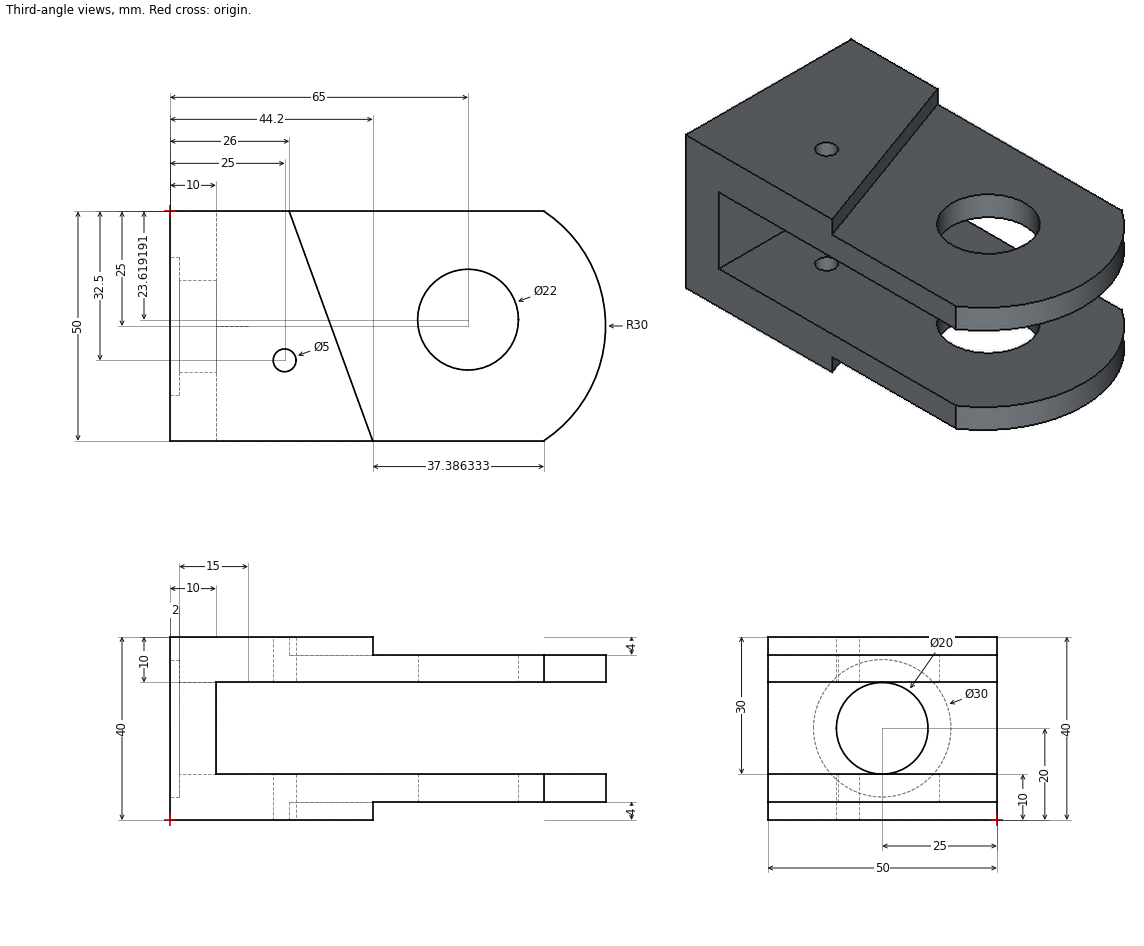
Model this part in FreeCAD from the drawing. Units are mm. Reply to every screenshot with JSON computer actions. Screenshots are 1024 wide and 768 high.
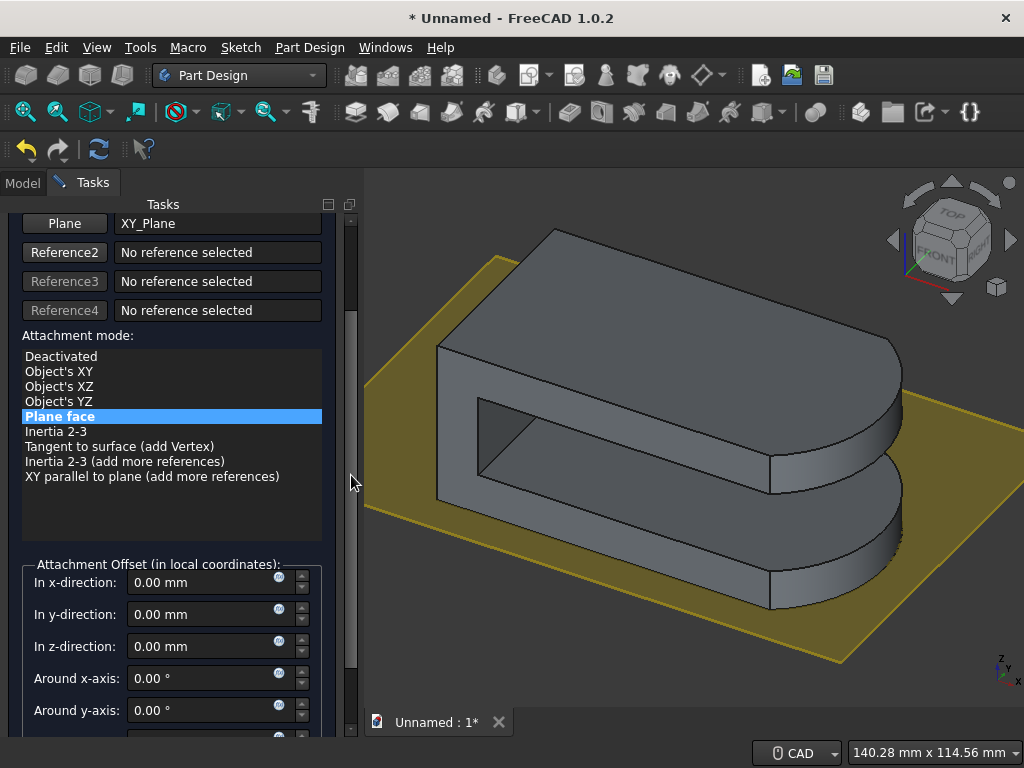
{"action": "triple_click", "coordinate": [210, 646]}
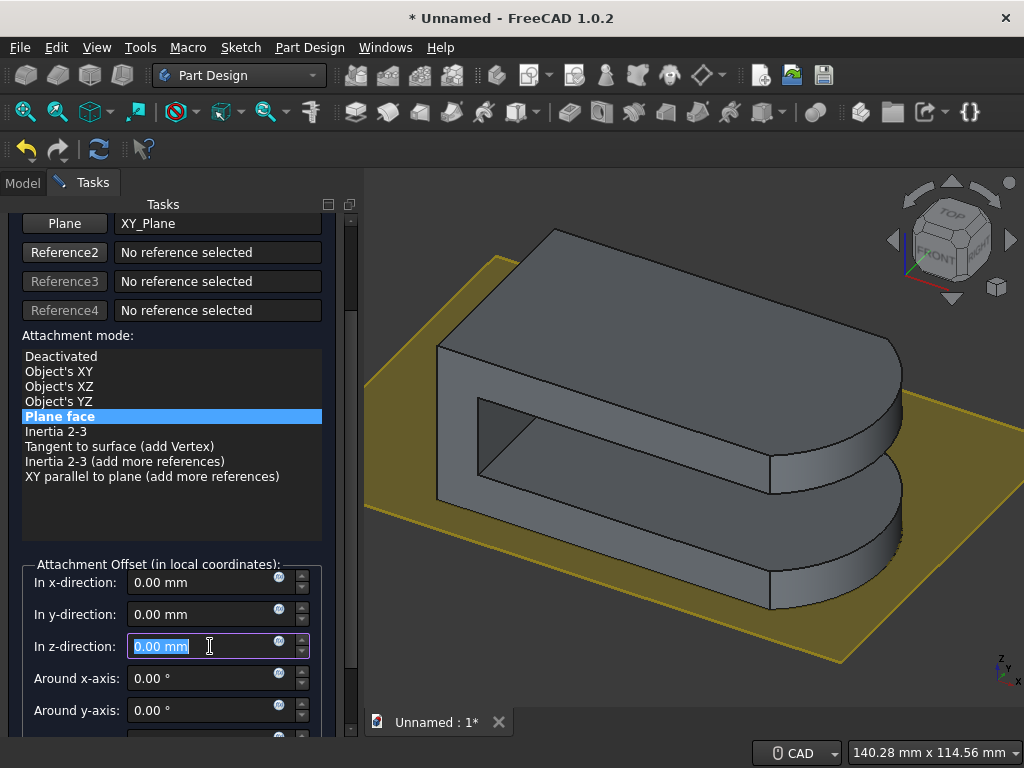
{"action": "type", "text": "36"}
{"action": "key", "text": "Tab"}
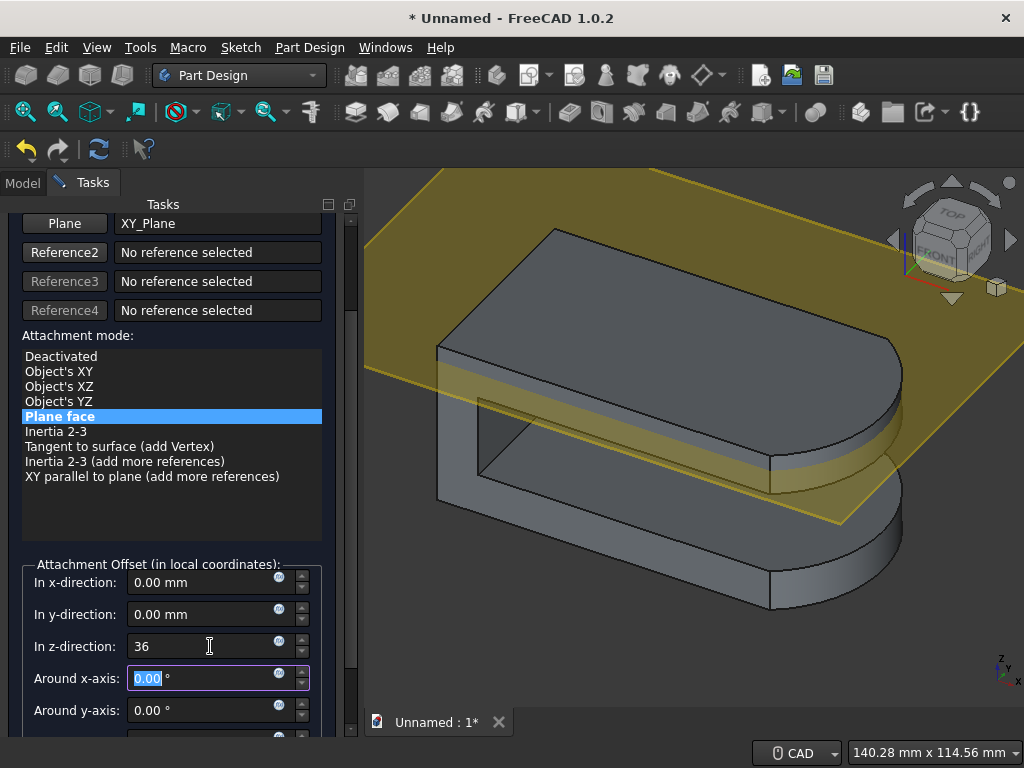
{"action": "scroll", "coordinate": [351, 475], "scroll_direction": "up", "scroll_amount": 3}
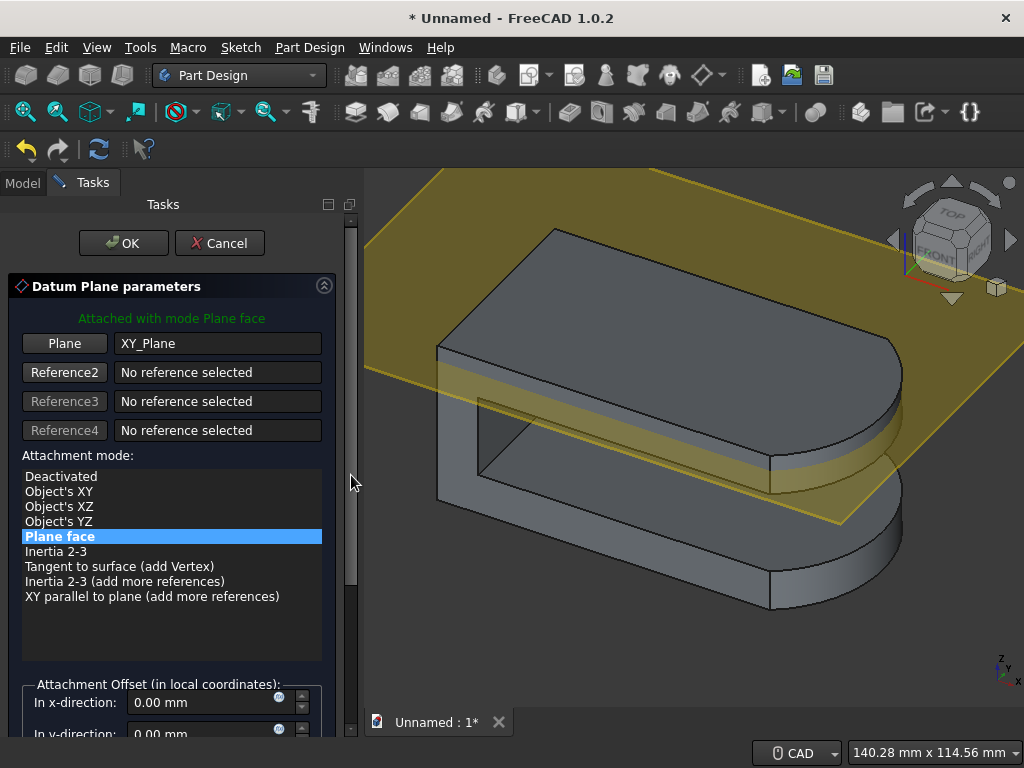
{"action": "left_click", "coordinate": [124, 243]}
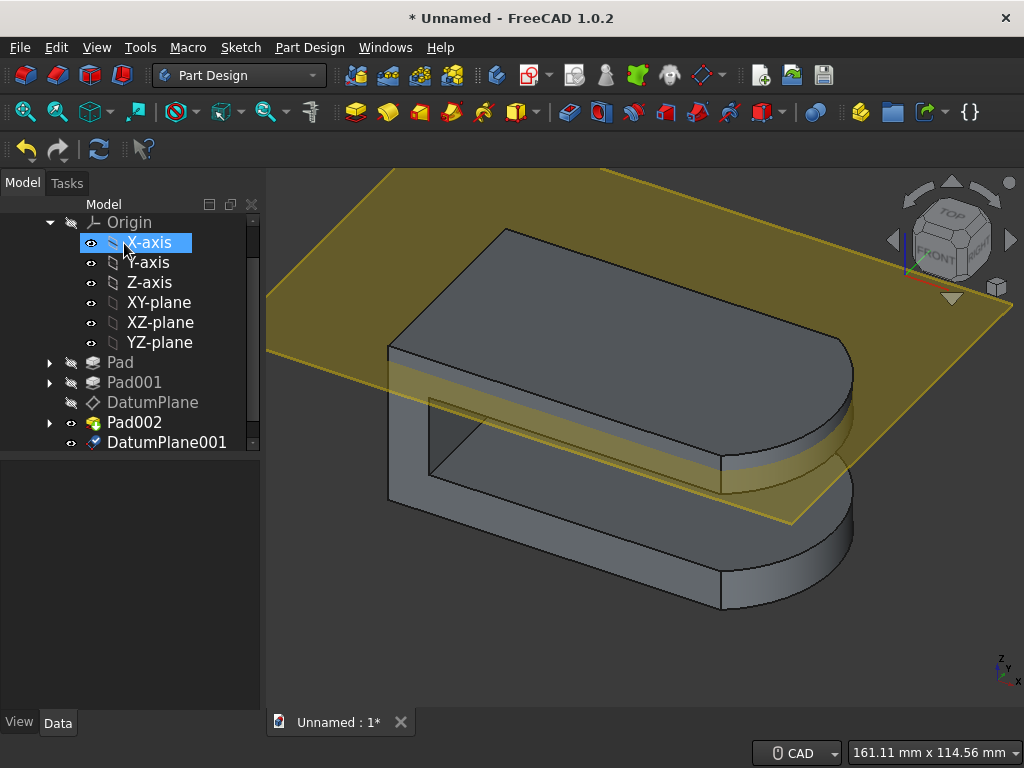
{"action": "left_click", "coordinate": [116, 443]}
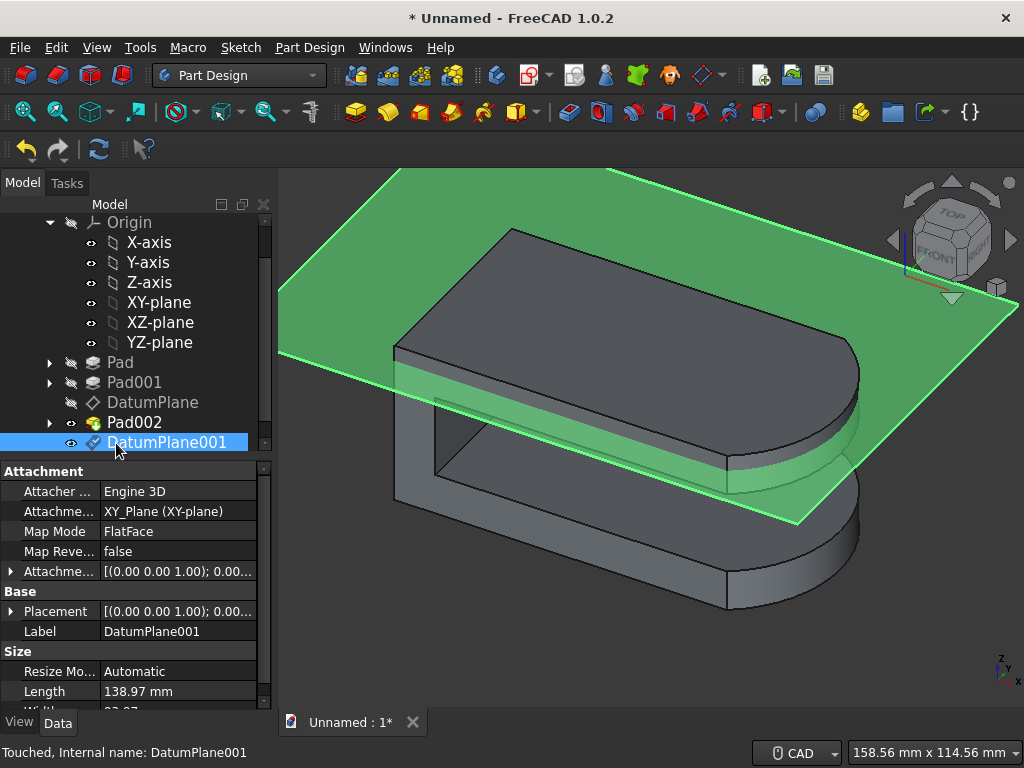
{"action": "left_click", "coordinate": [530, 76]}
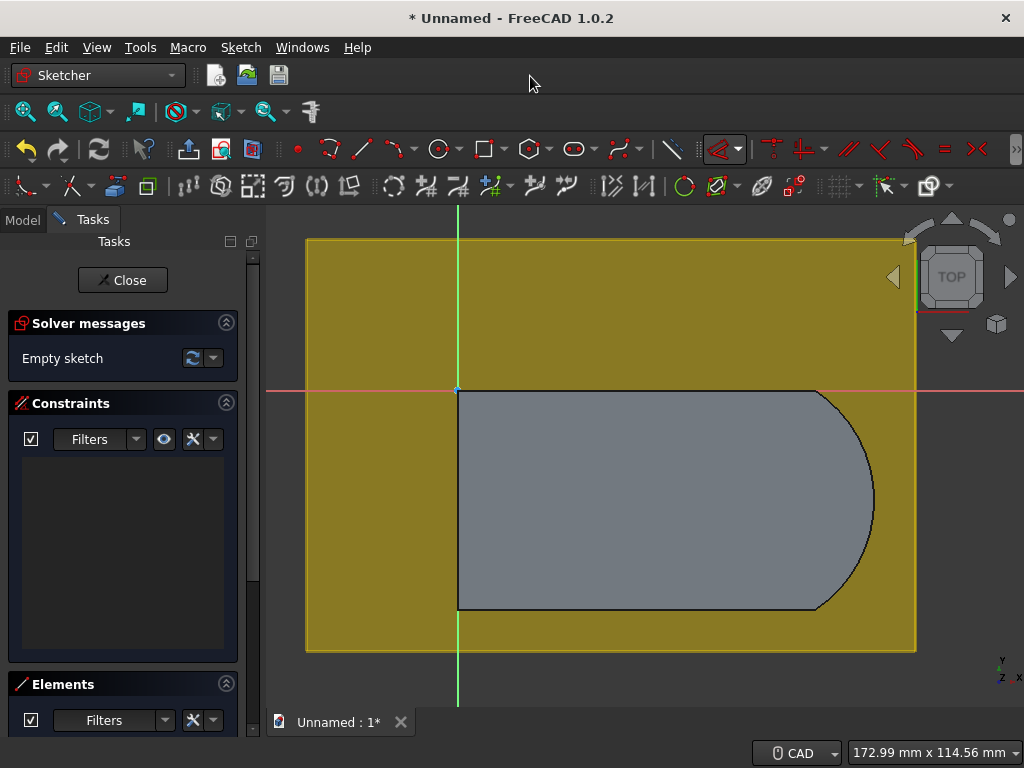
{"action": "left_click", "coordinate": [254, 150]}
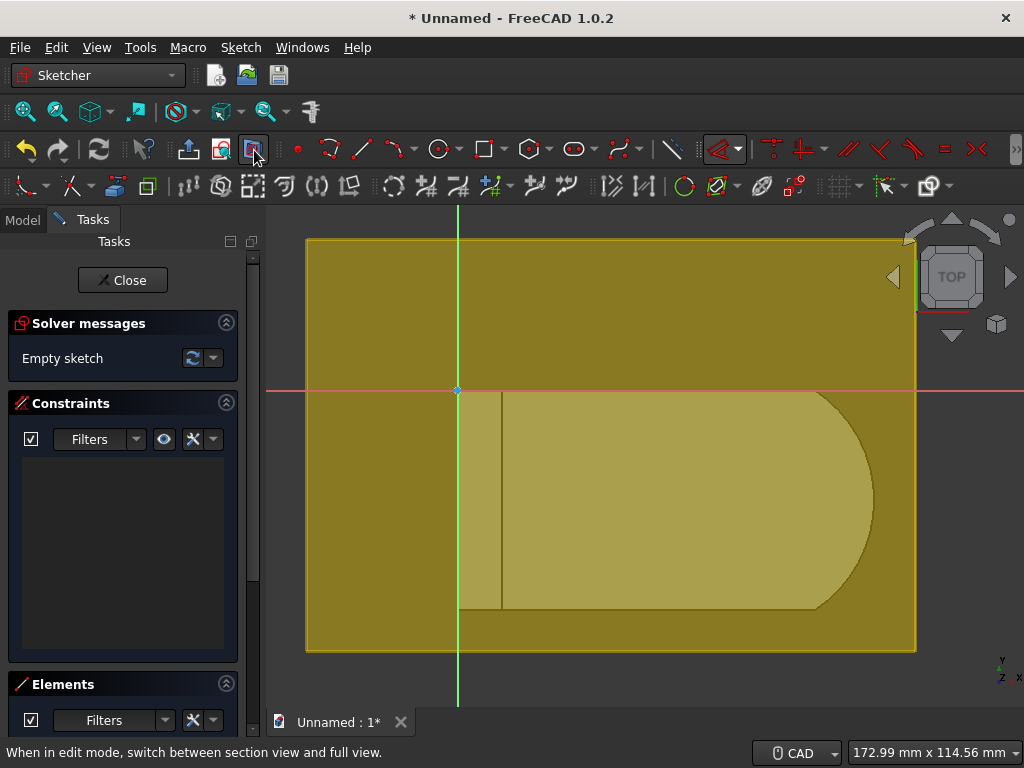
{"action": "scroll", "coordinate": [294, 256], "scroll_direction": "down", "scroll_amount": 1}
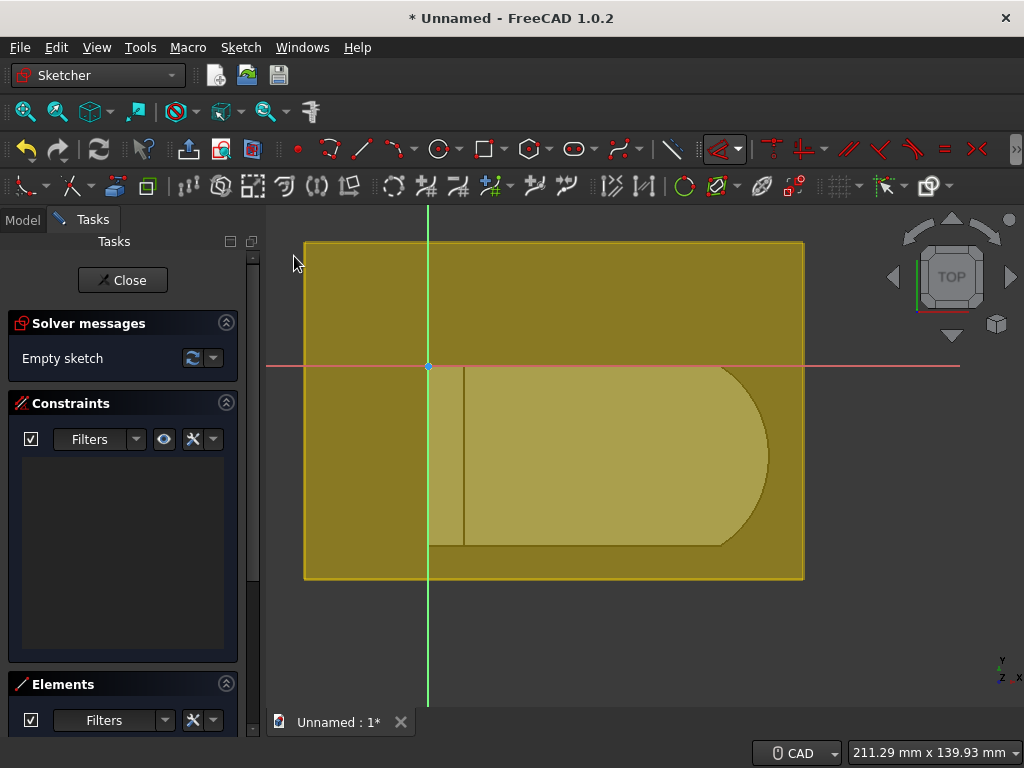
{"action": "left_click", "coordinate": [330, 150]}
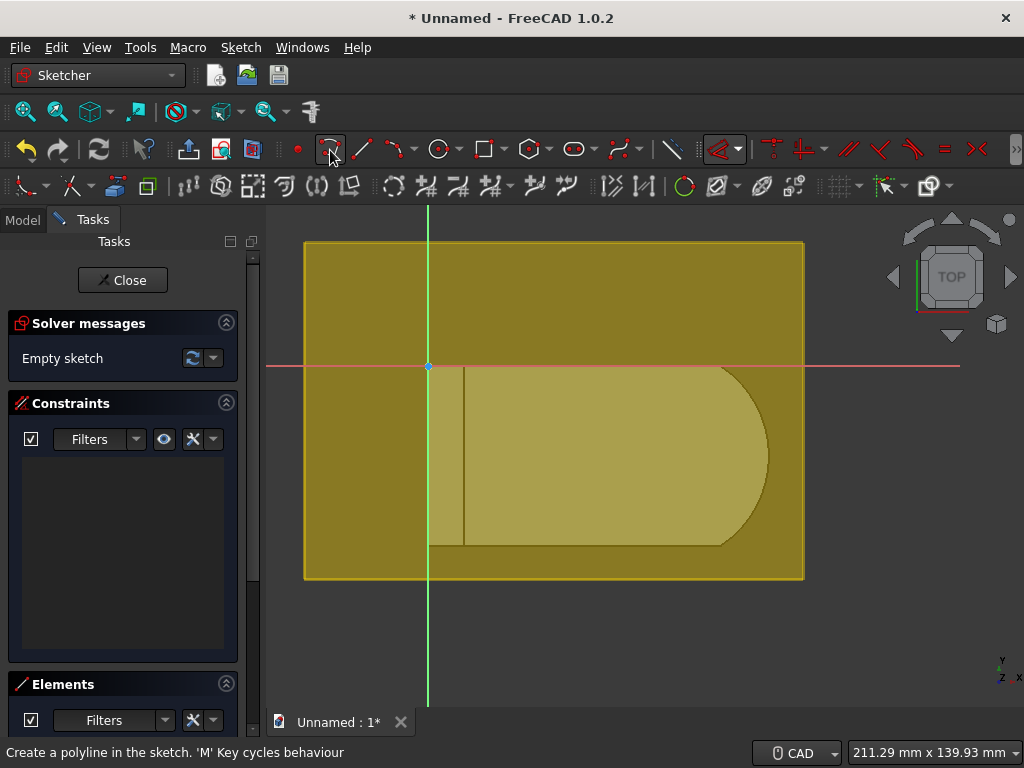
{"action": "left_click", "coordinate": [721, 366]}
{"action": "left_click", "coordinate": [521, 375]}
{"action": "left_click", "coordinate": [587, 546]}
{"action": "left_click", "coordinate": [721, 546]}
{"action": "right_click", "coordinate": [721, 546]}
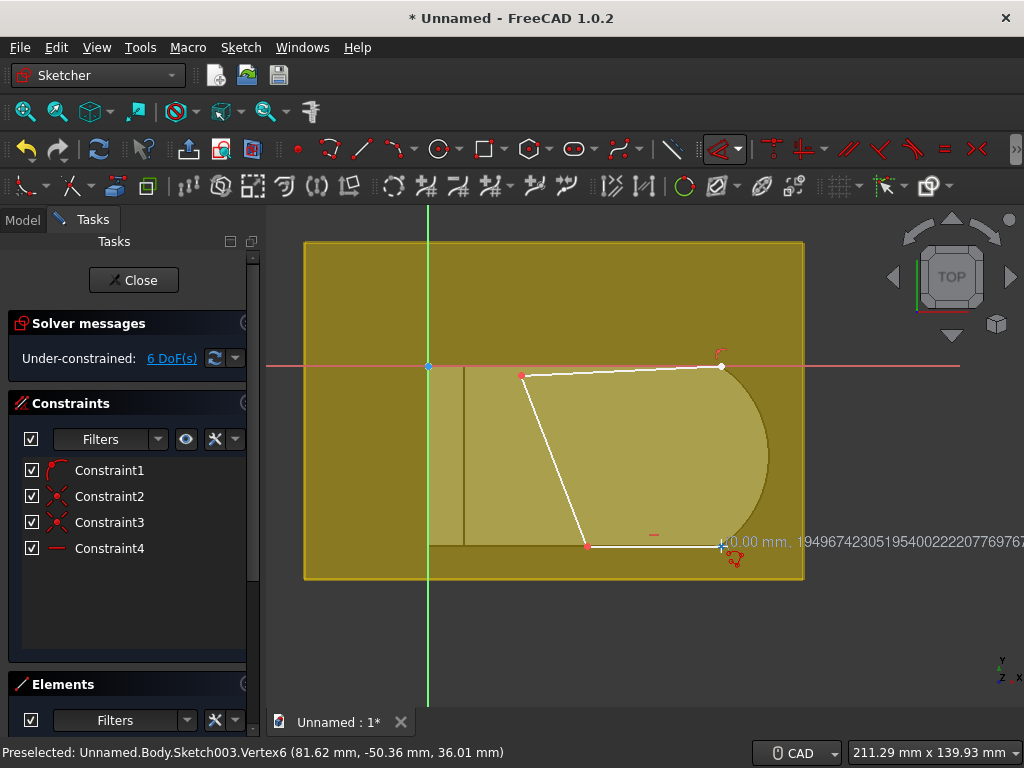
{"action": "left_click", "coordinate": [394, 150]}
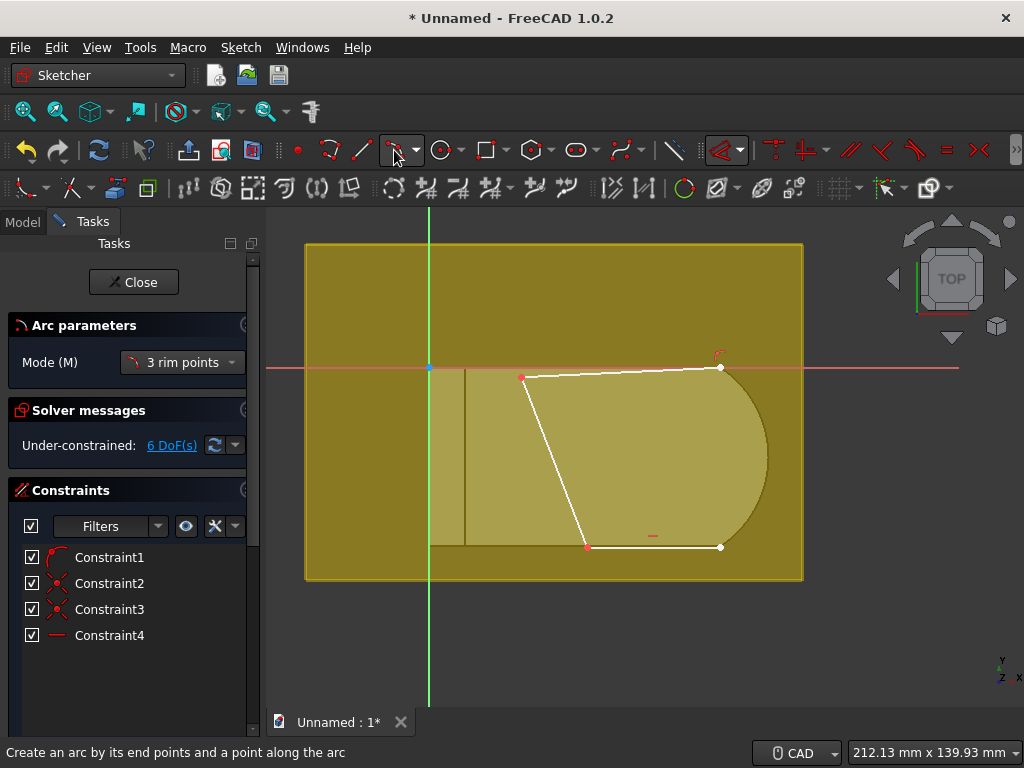
{"action": "left_click", "coordinate": [721, 548]}
{"action": "left_click", "coordinate": [721, 368]}
{"action": "left_click", "coordinate": [769, 457]}
{"action": "key", "text": "Escape"}